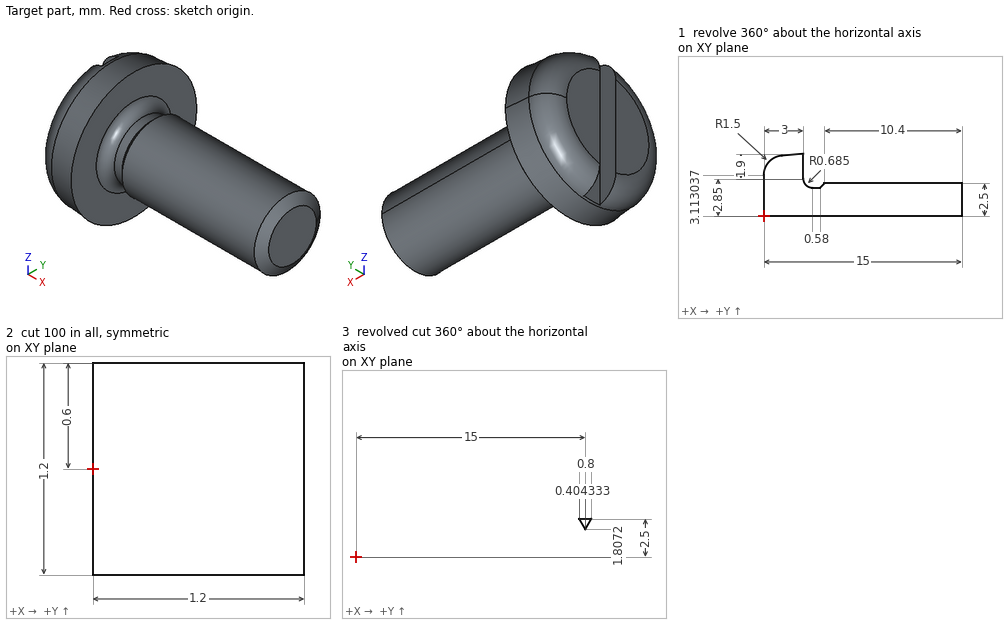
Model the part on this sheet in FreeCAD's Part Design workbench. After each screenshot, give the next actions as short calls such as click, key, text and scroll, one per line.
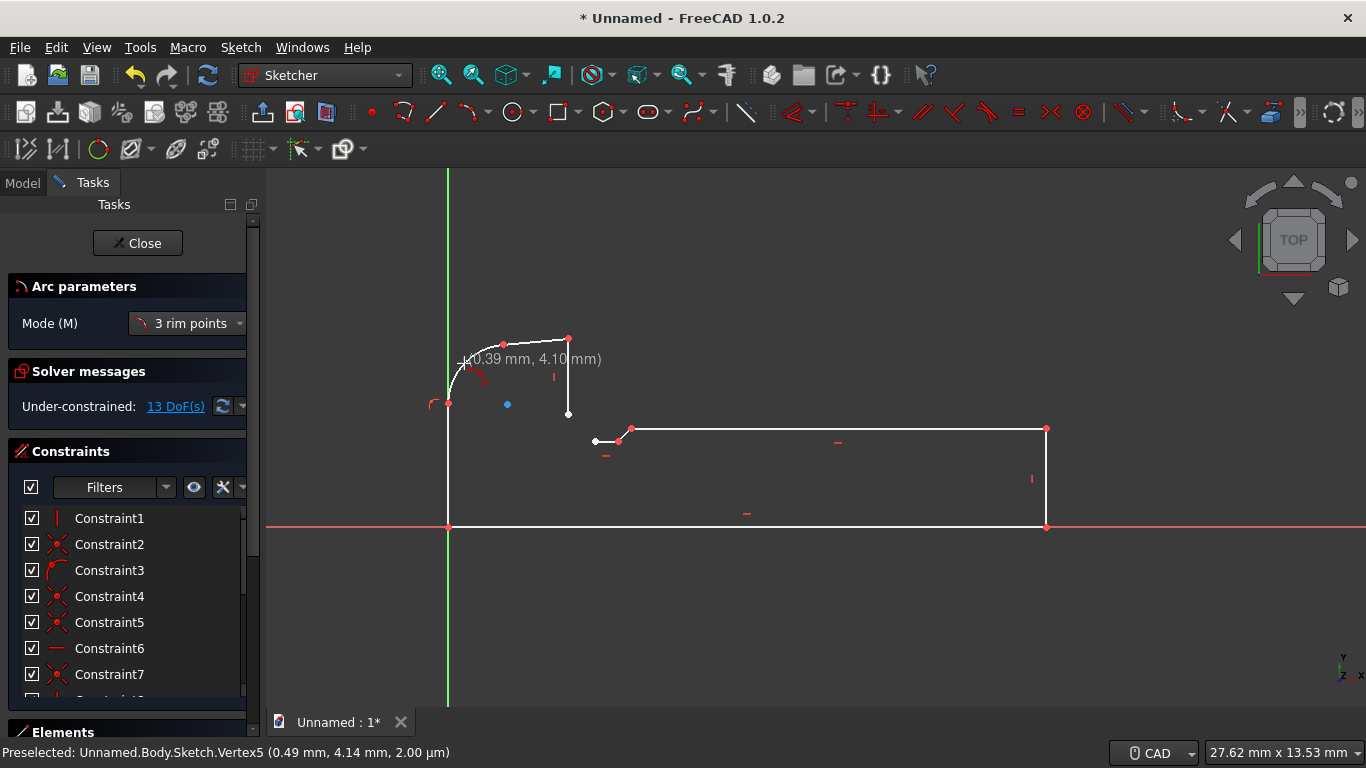
scroll(595, 441, up, 2)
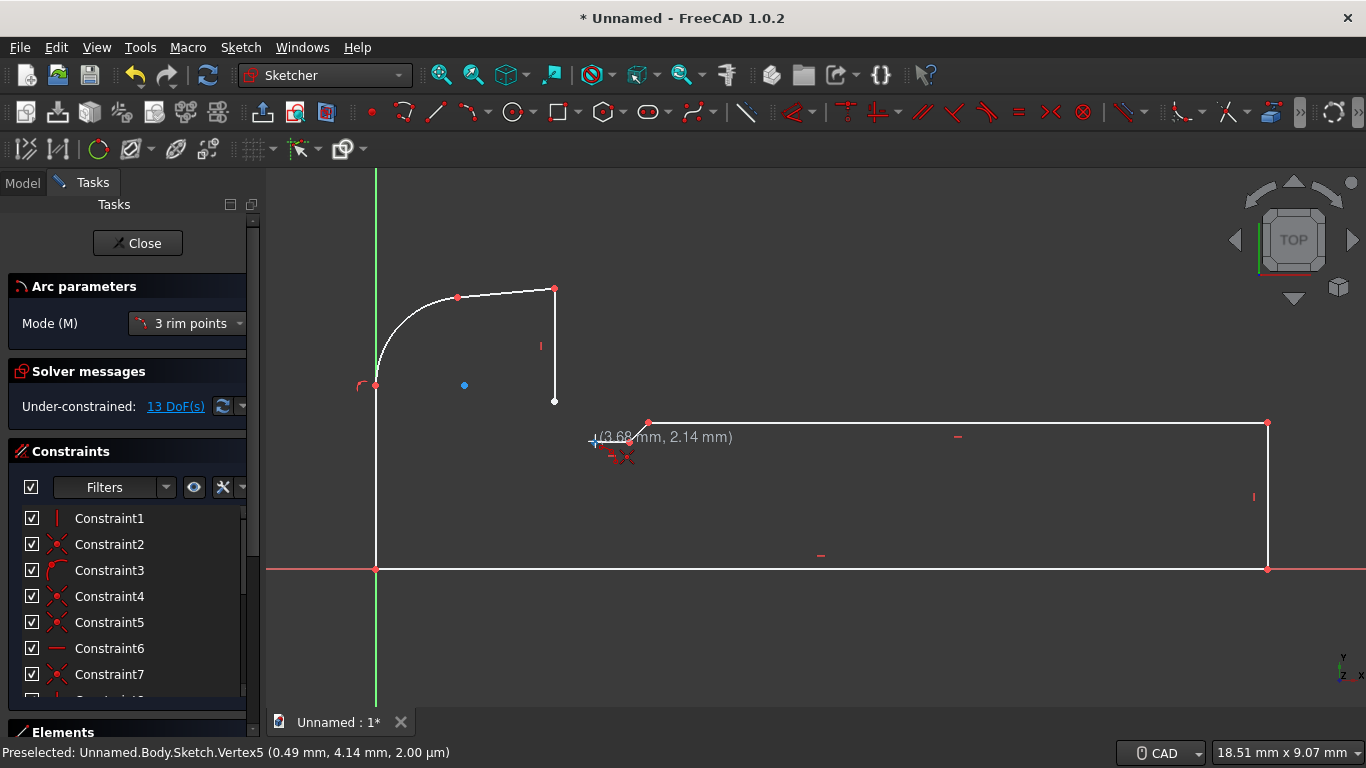
click(595, 442)
click(555, 402)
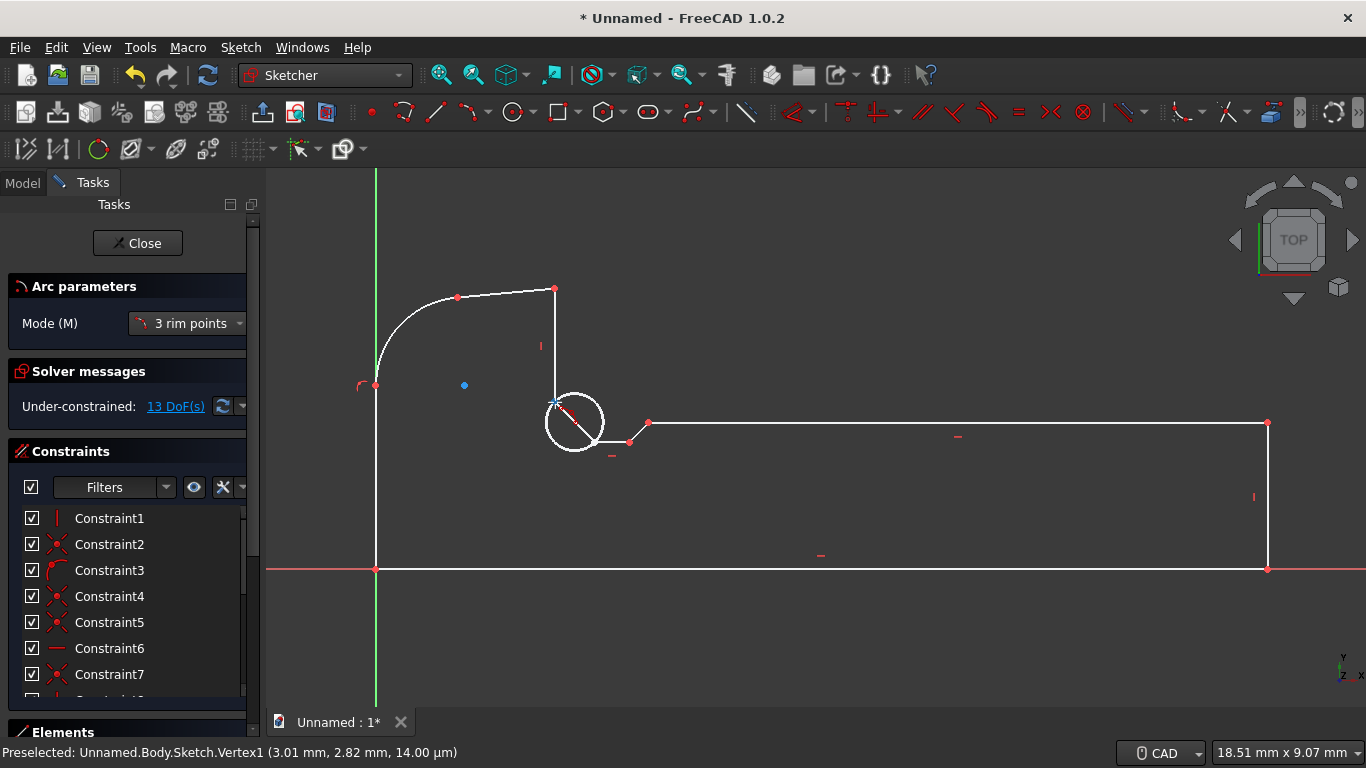
scroll(566, 429, up, 2)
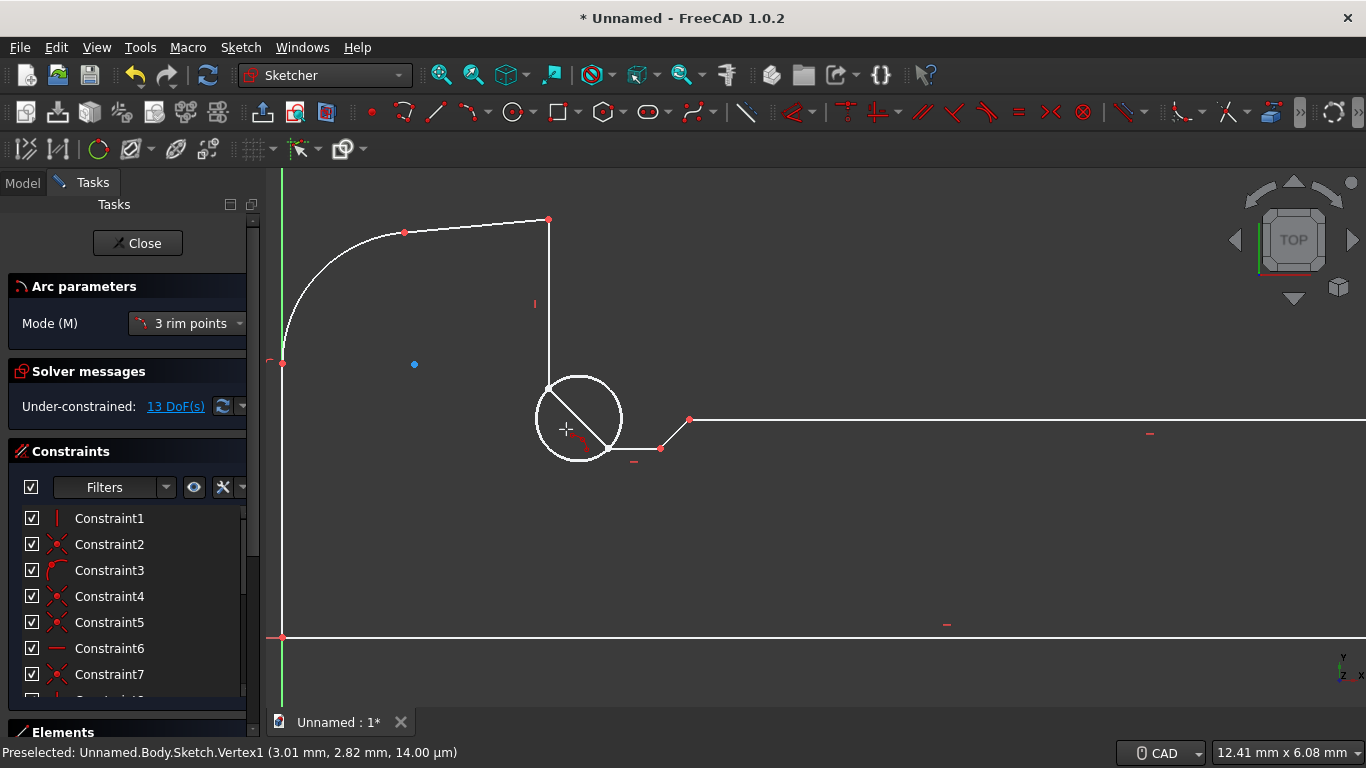
click(566, 428)
key(Escape)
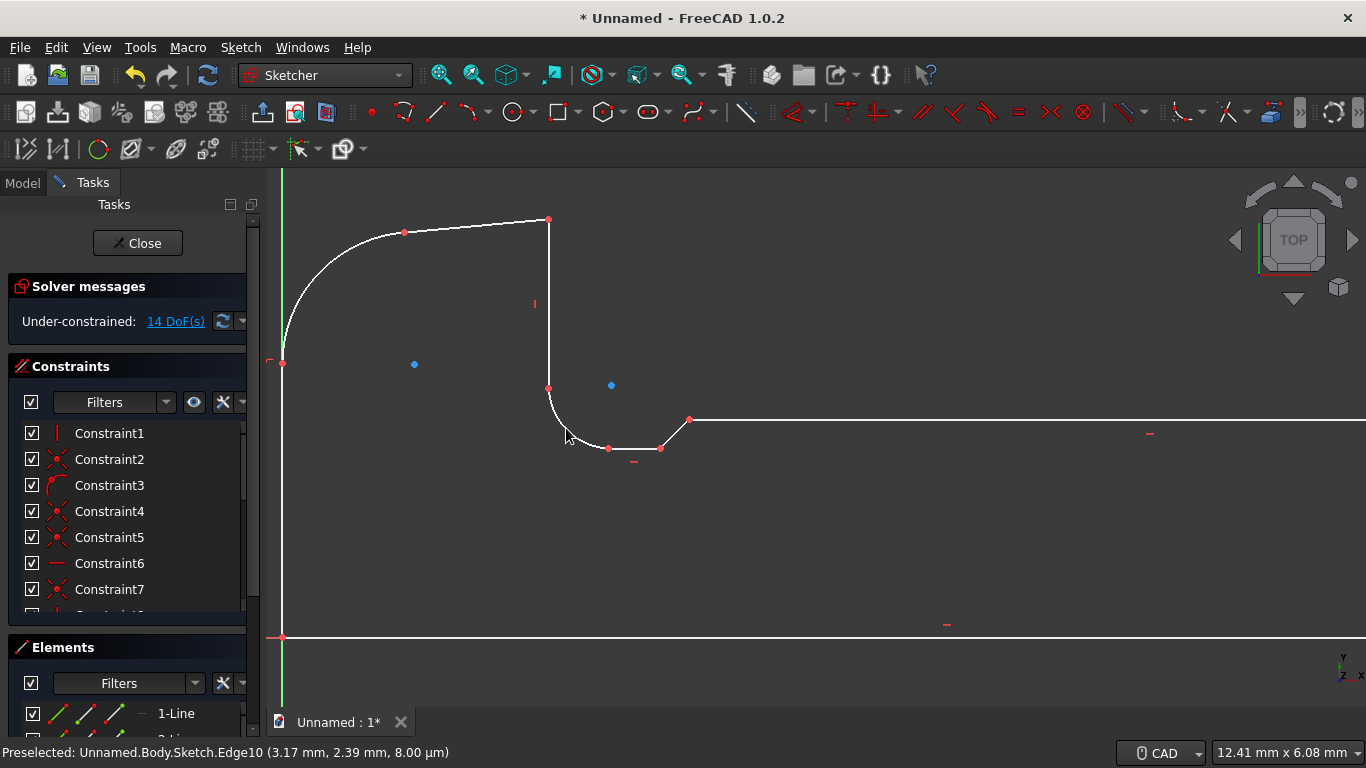
click(549, 338)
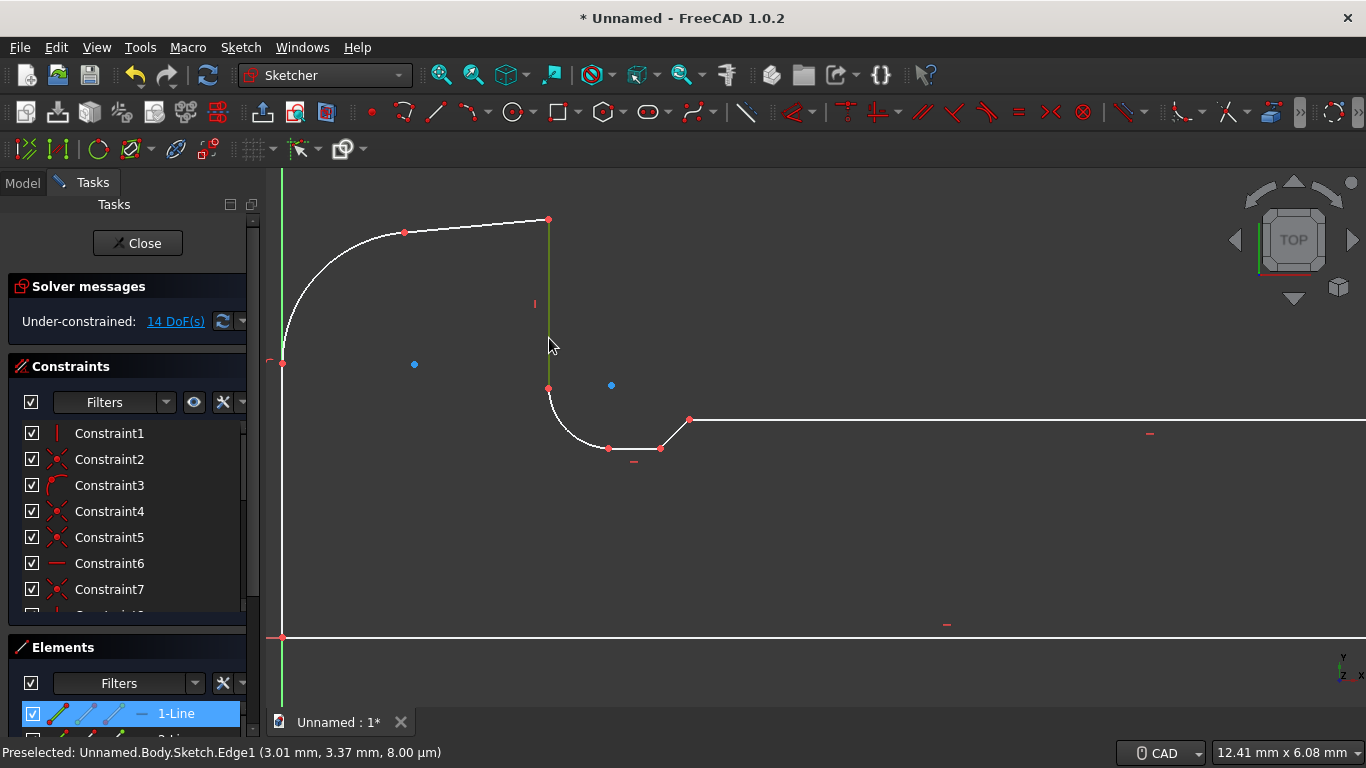
click(556, 415)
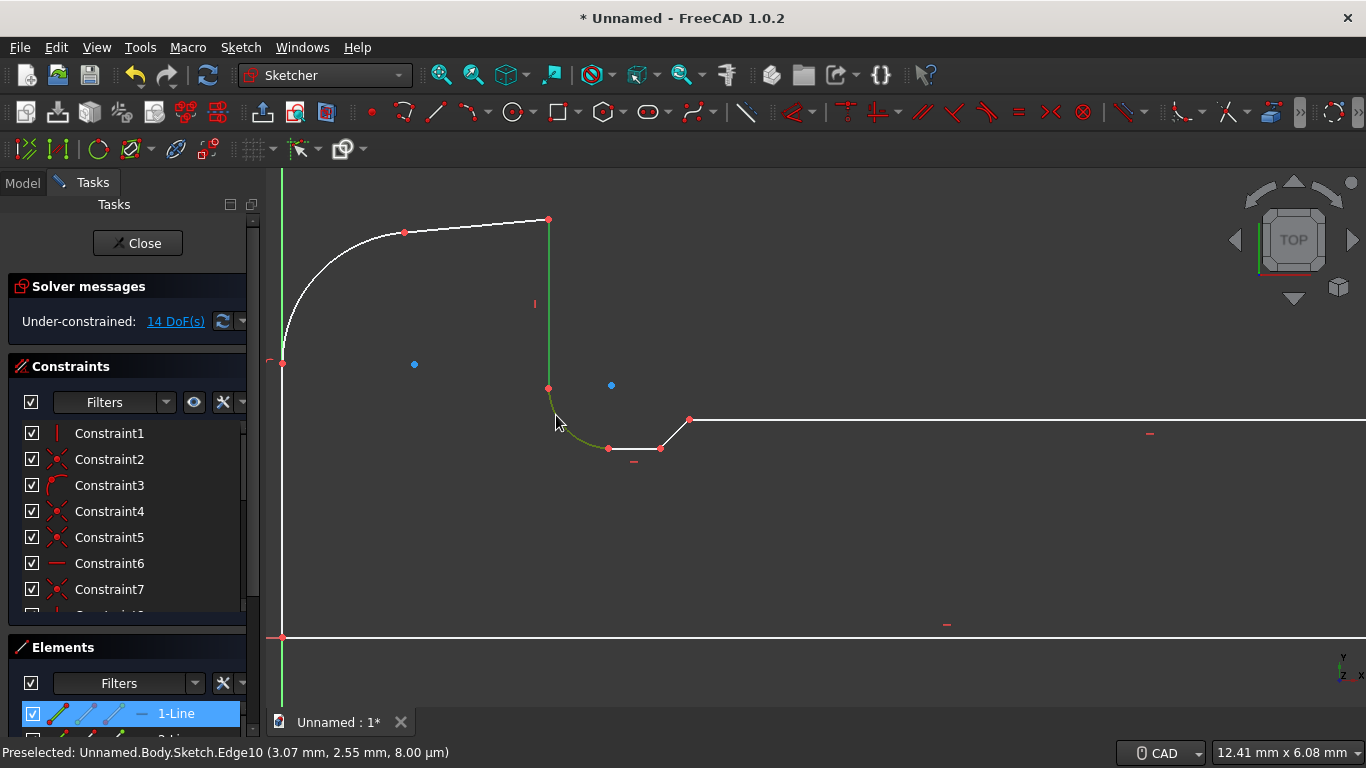
key(t)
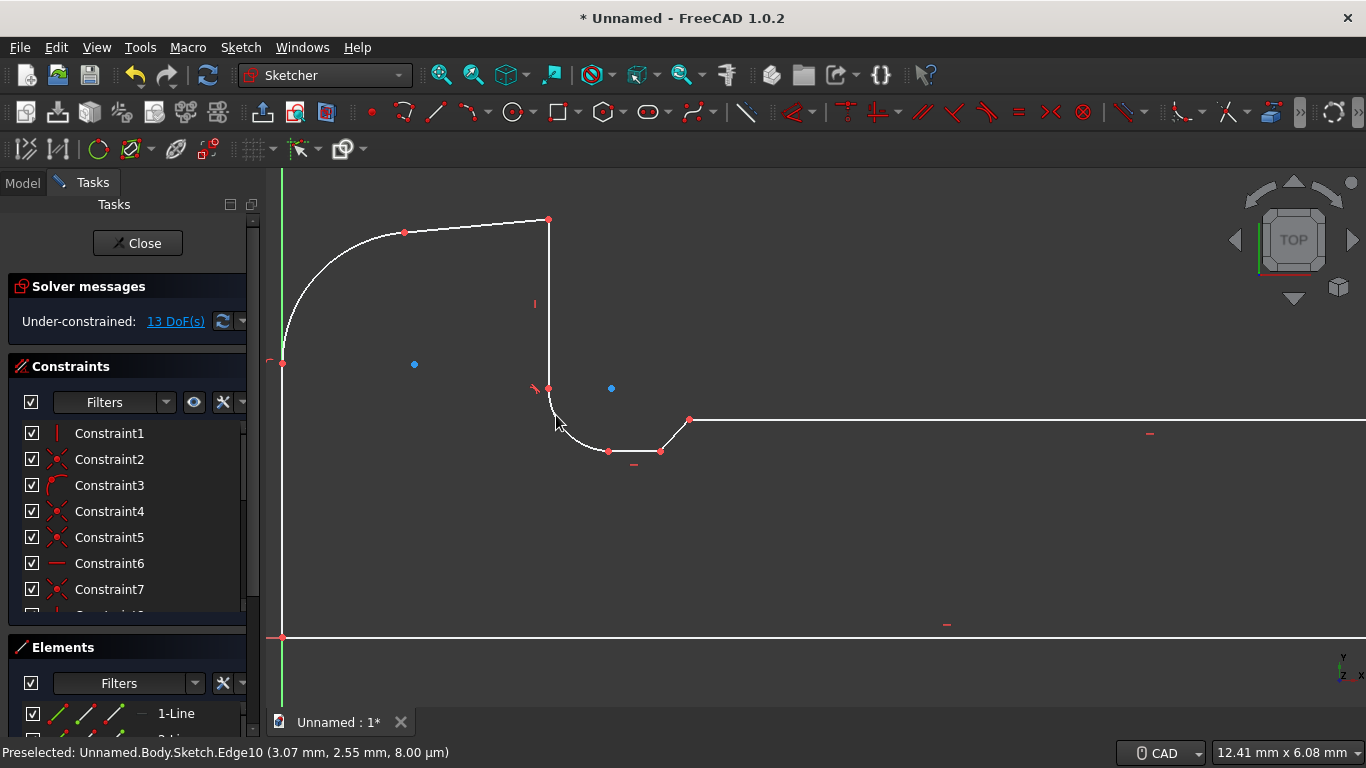
click(505, 223)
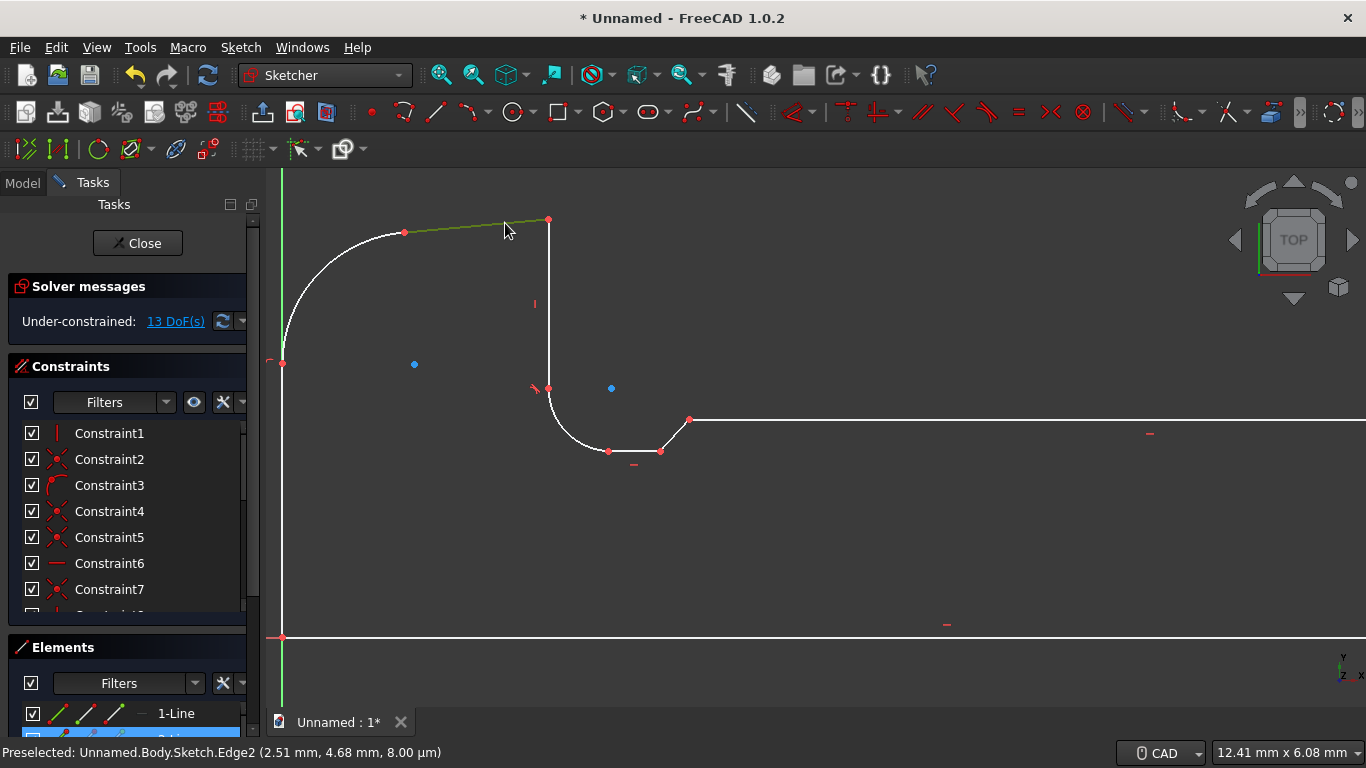
click(348, 250)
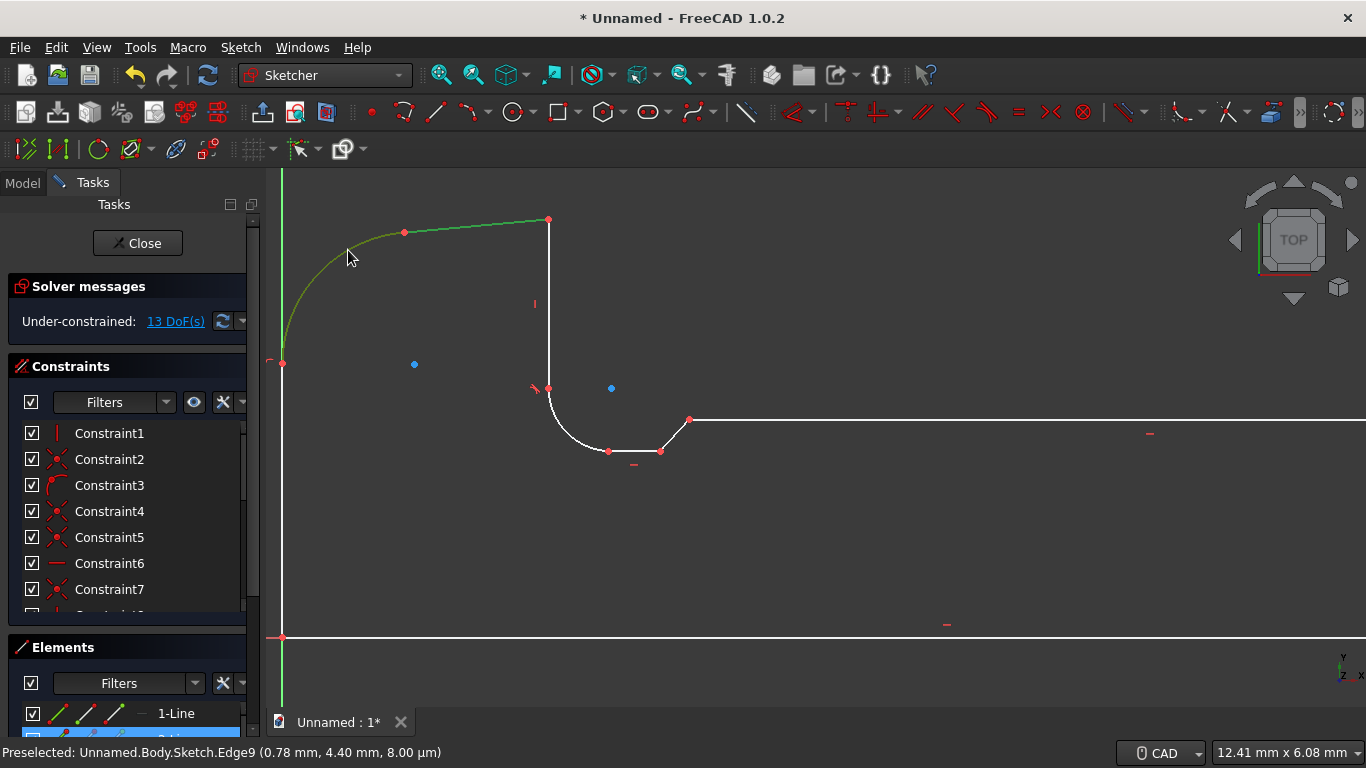
key(t)